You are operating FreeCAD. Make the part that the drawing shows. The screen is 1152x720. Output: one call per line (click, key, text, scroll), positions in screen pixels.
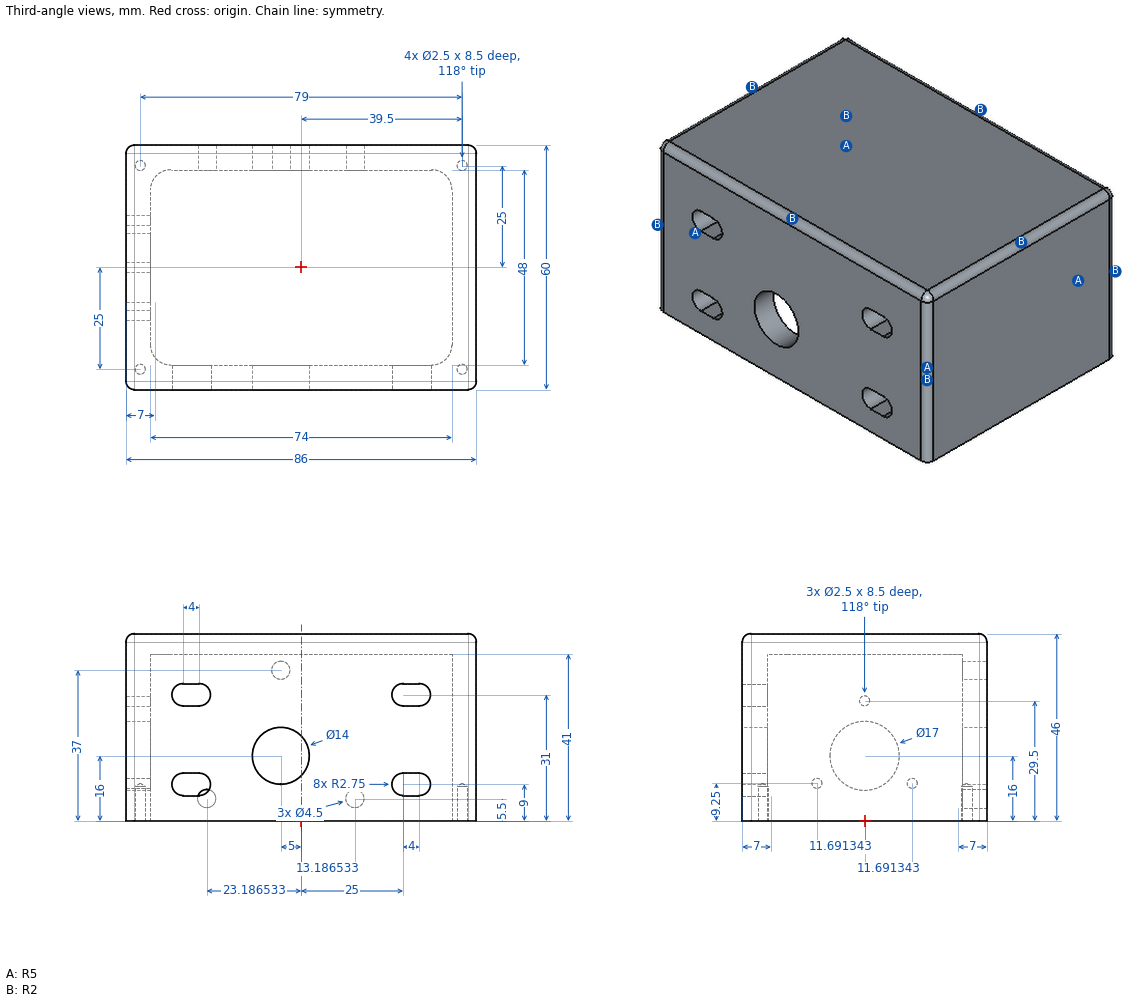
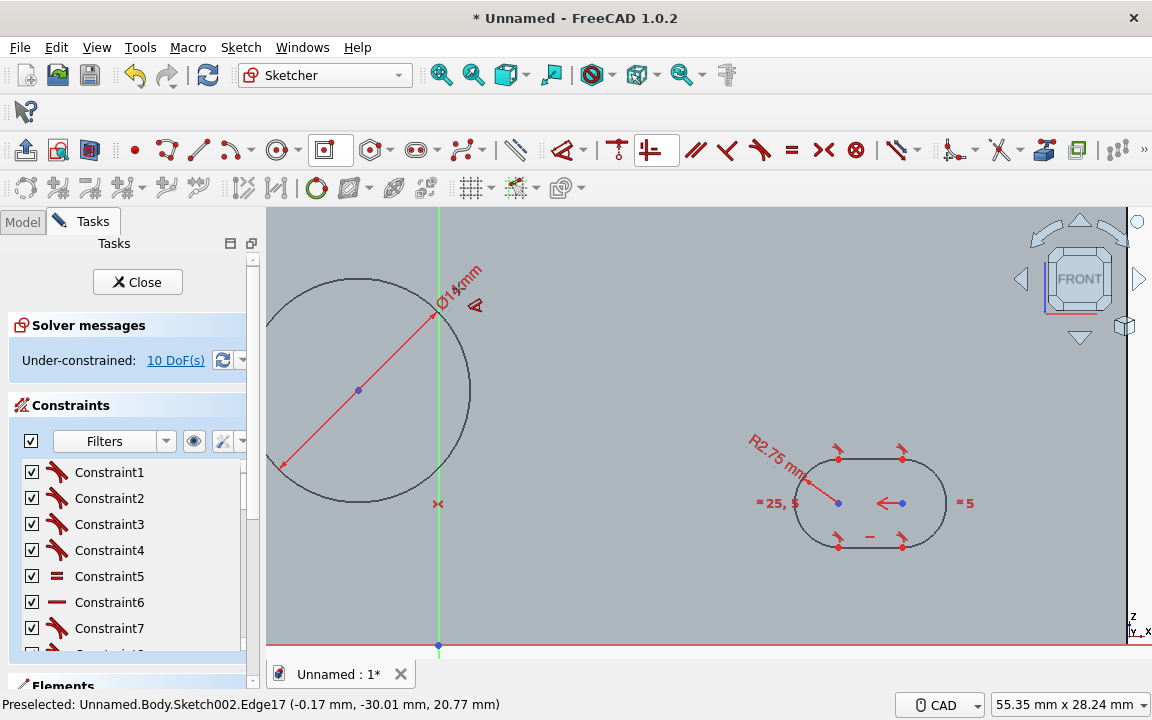
click(858, 459)
click(871, 493)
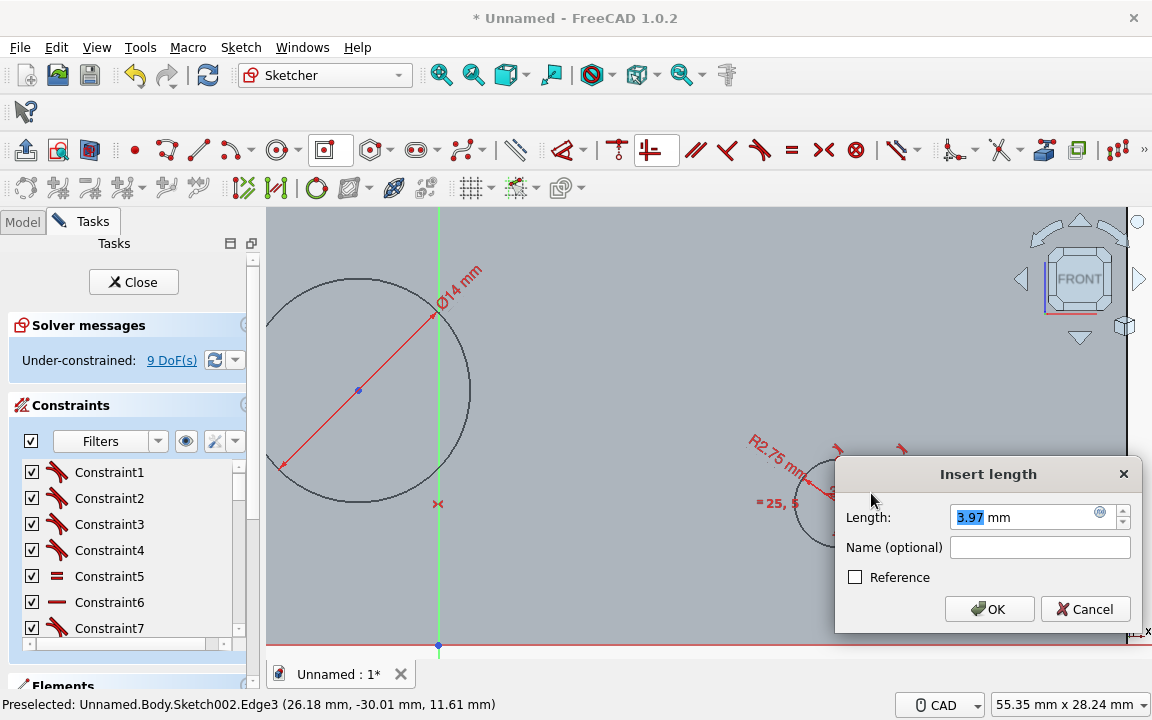
text(4)
key(Return)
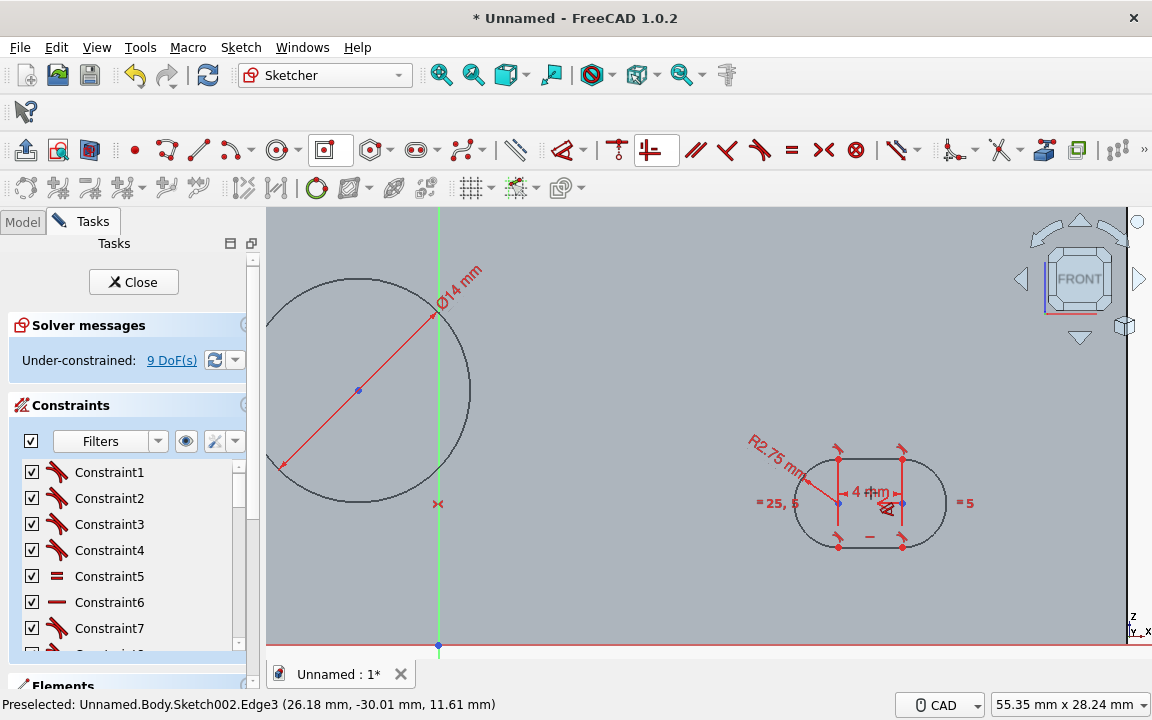
scroll(805, 480, down, 4)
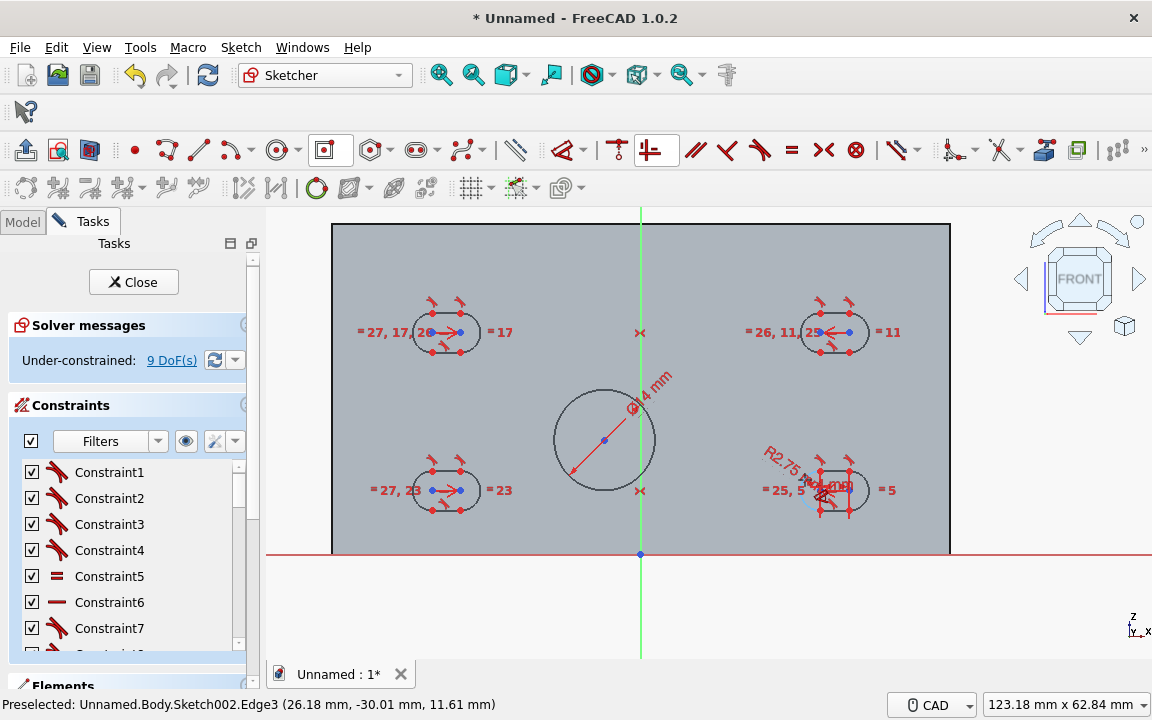
scroll(829, 313, up, 3)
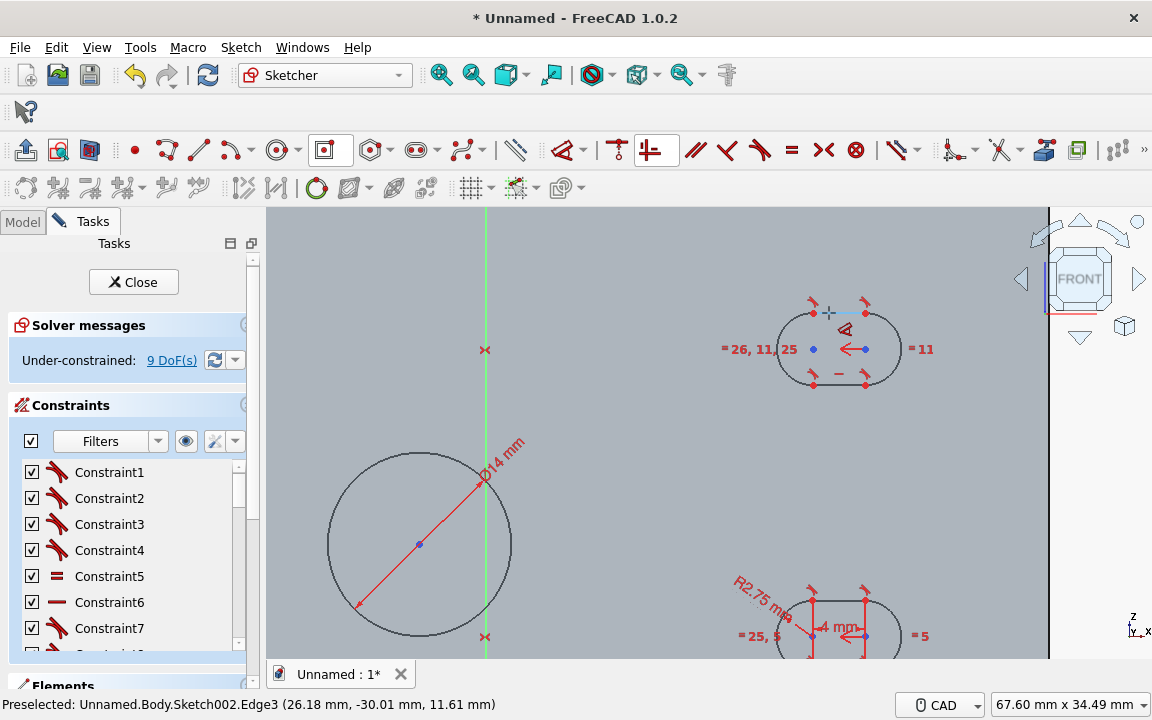
click(829, 313)
click(839, 279)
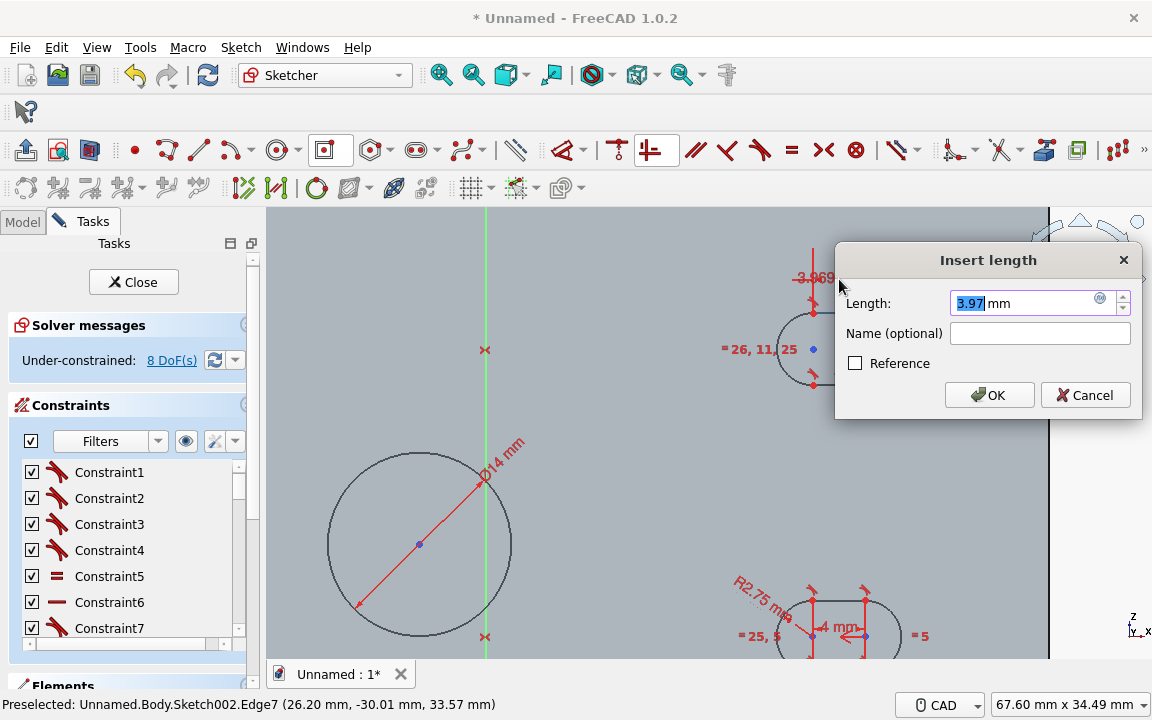
text(4)
key(Return)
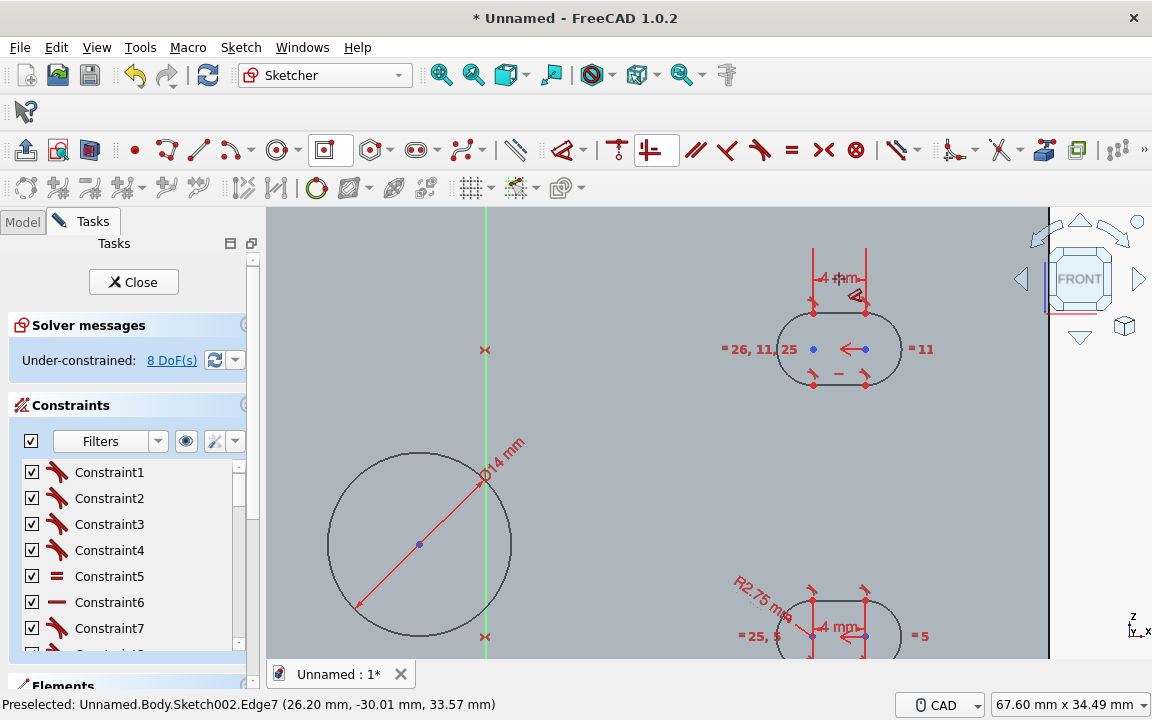
scroll(829, 313, down, 3)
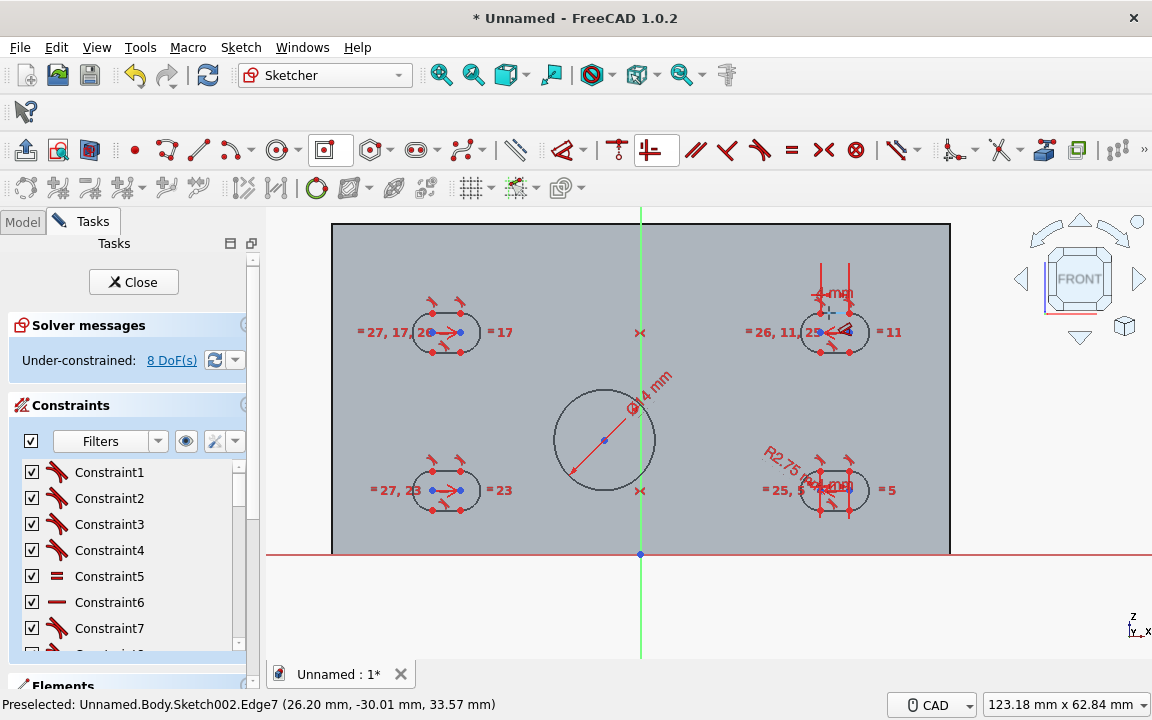
scroll(441, 313, up, 3)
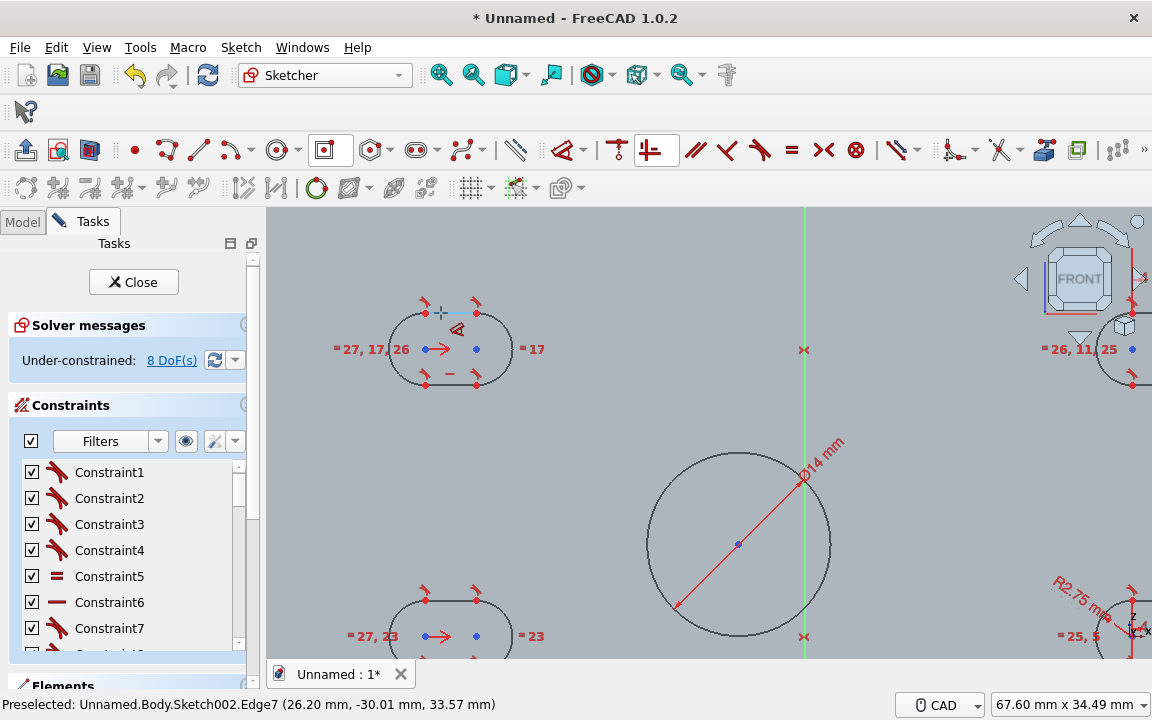
click(440, 313)
click(451, 279)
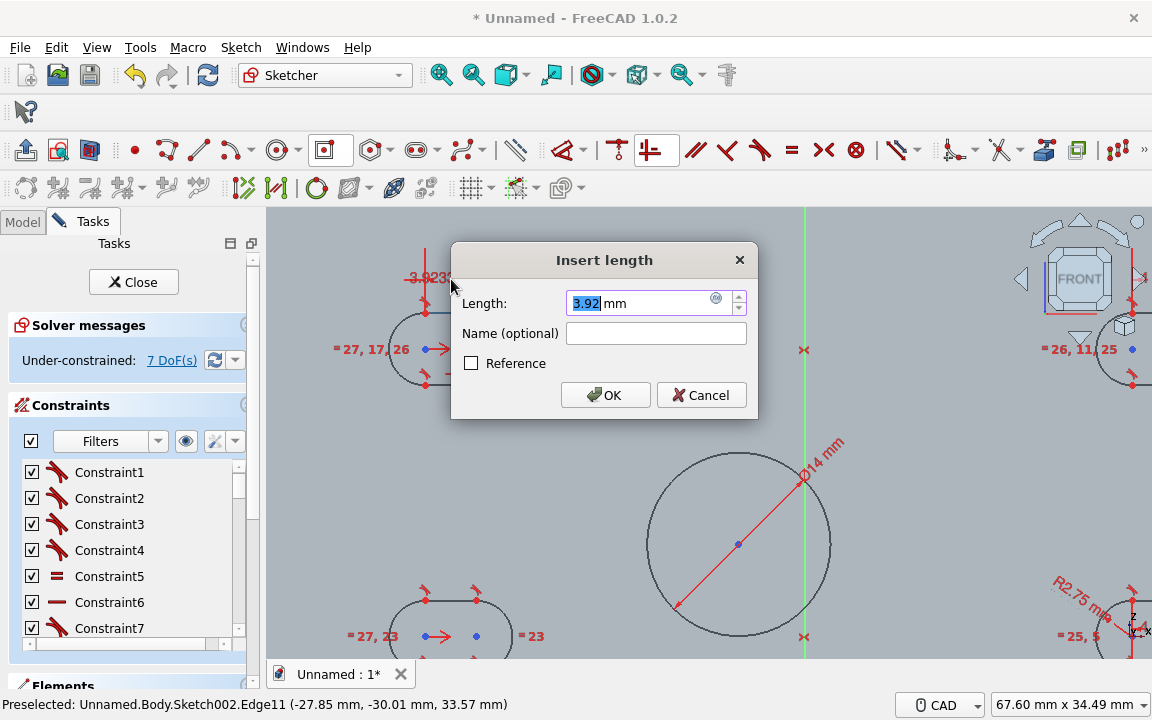
text(4)
key(Return)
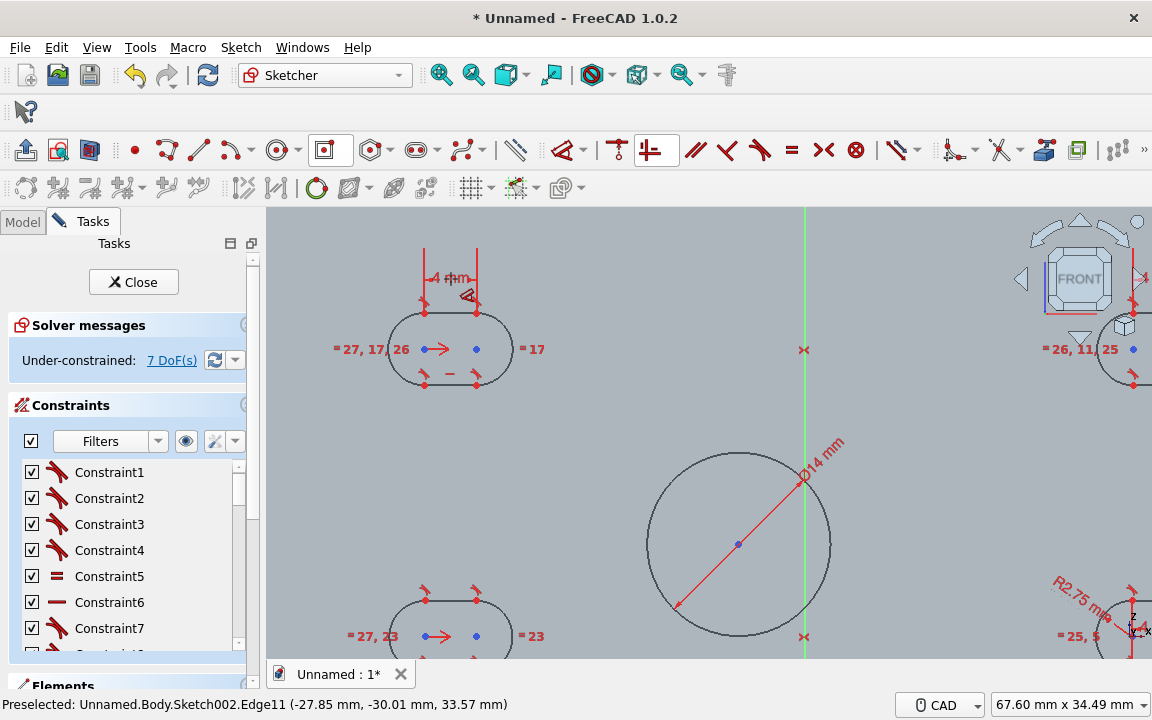
click(441, 601)
click(451, 567)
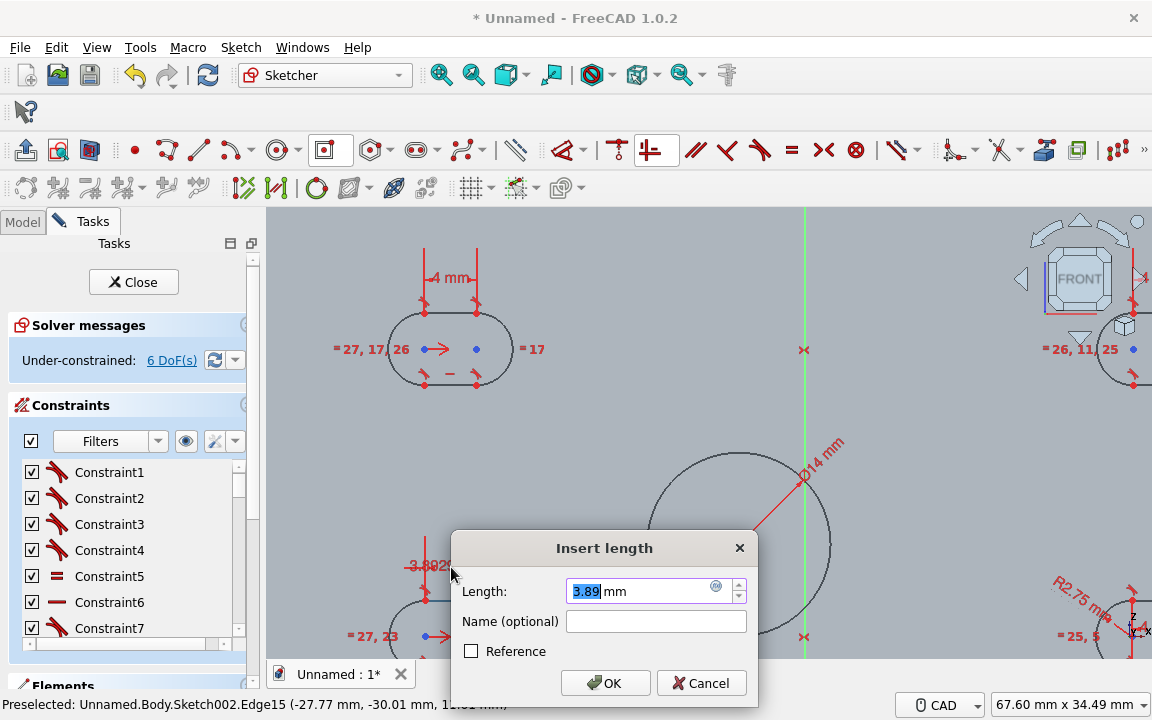
text(4)
key(Return)